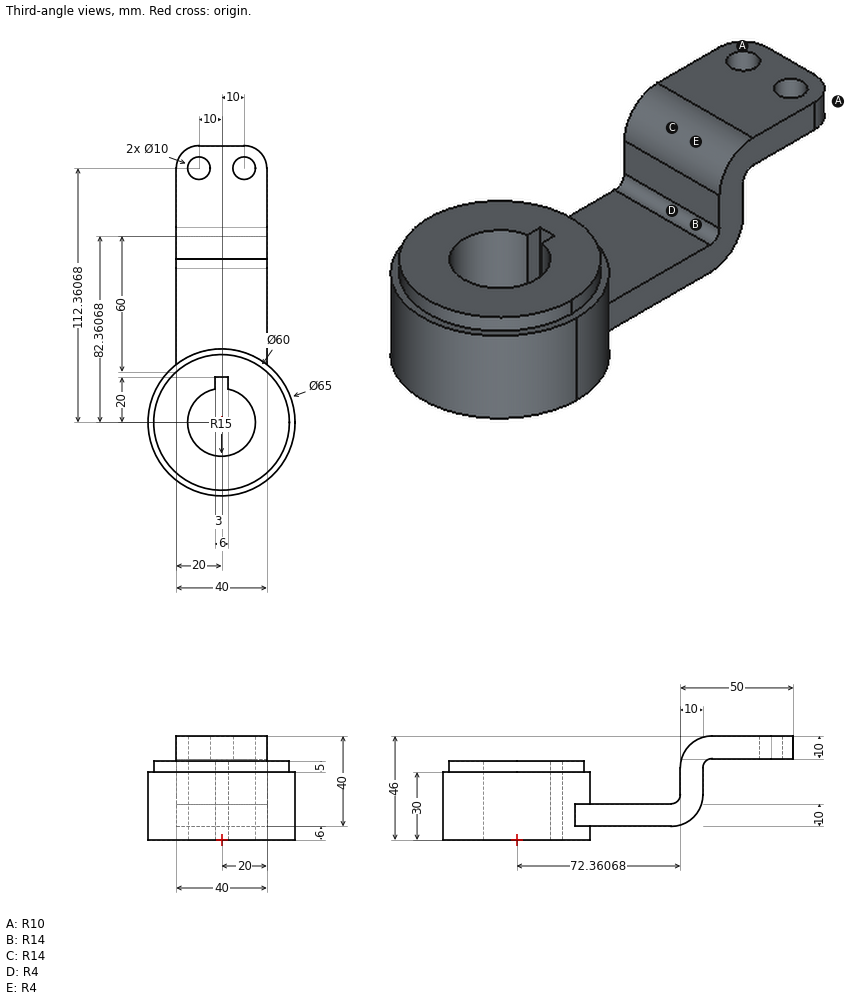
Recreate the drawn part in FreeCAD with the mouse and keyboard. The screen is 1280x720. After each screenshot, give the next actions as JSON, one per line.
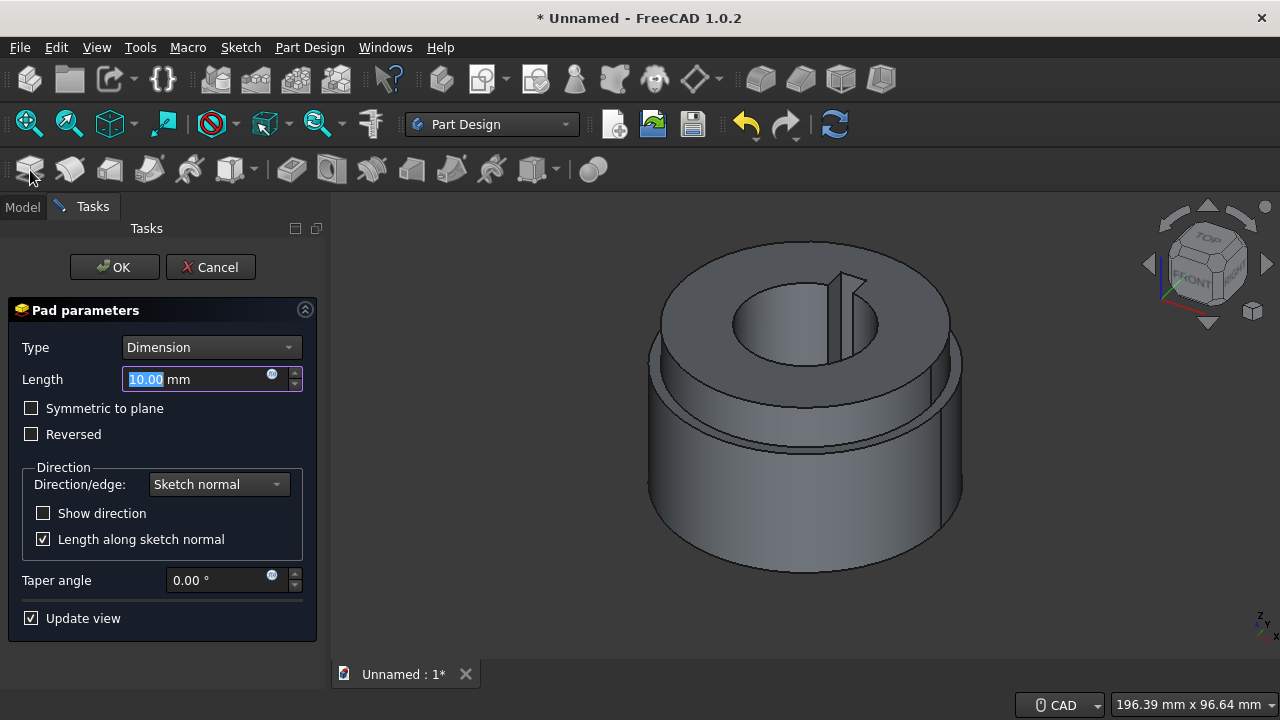
{"action": "type", "text": "5"}
{"action": "key", "text": "Tab"}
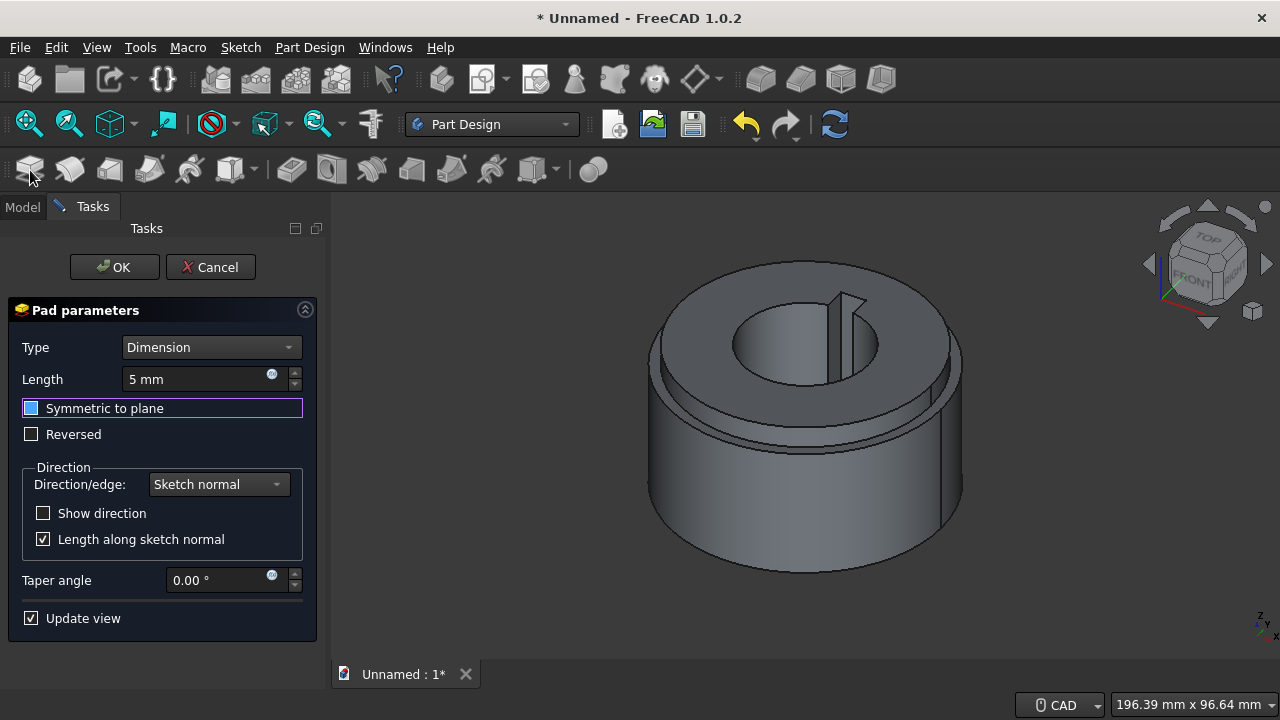
{"action": "left_click", "coordinate": [115, 267]}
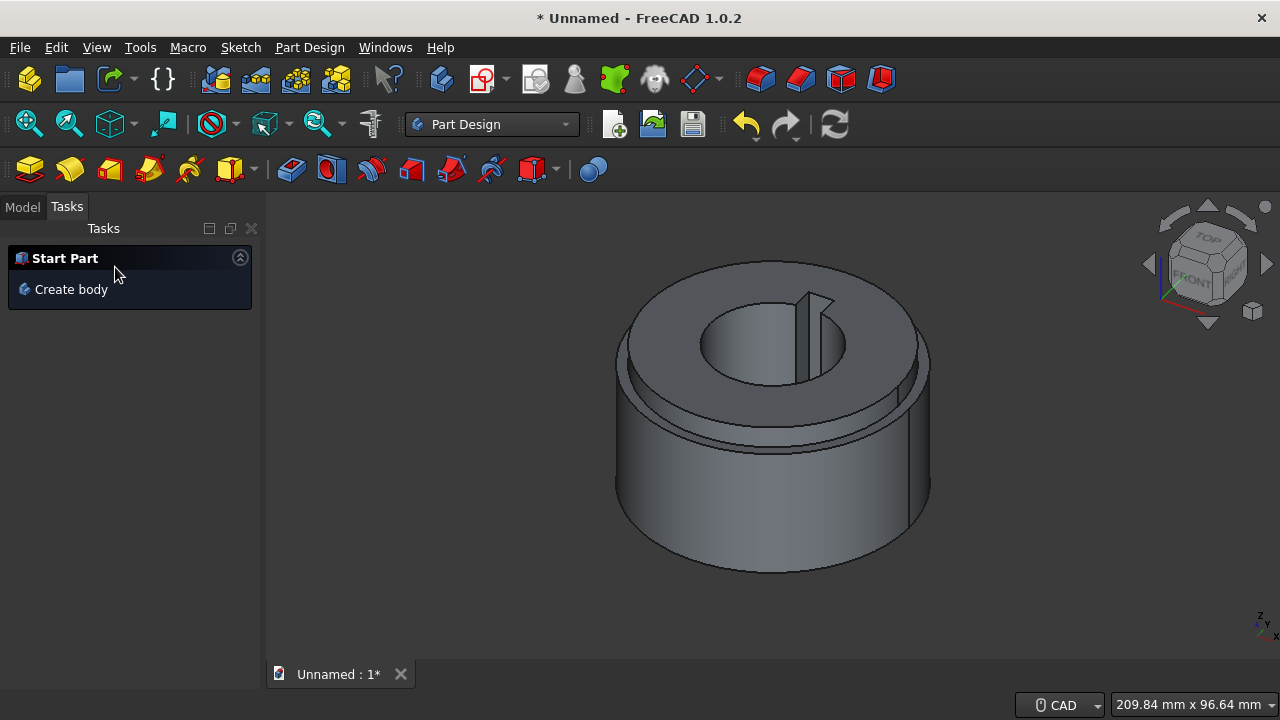
{"action": "left_click", "coordinate": [23, 206]}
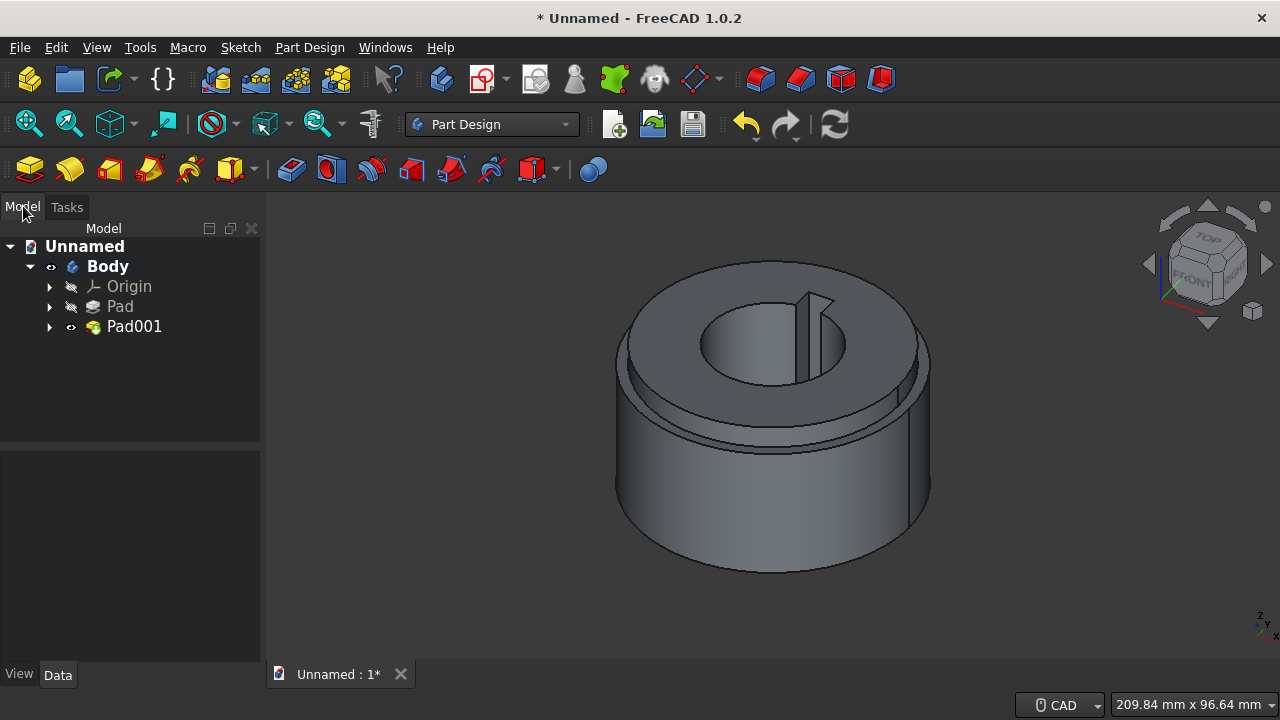
{"action": "left_click", "coordinate": [50, 287]}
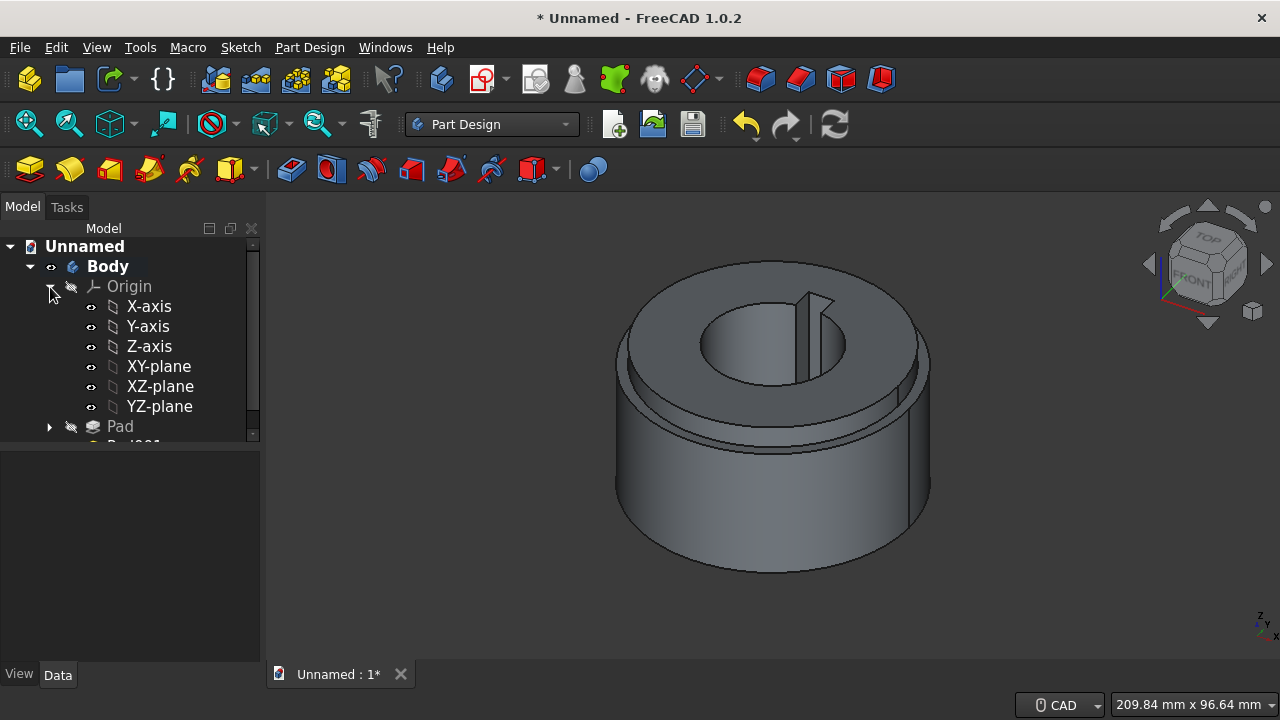
{"action": "left_click", "coordinate": [136, 367]}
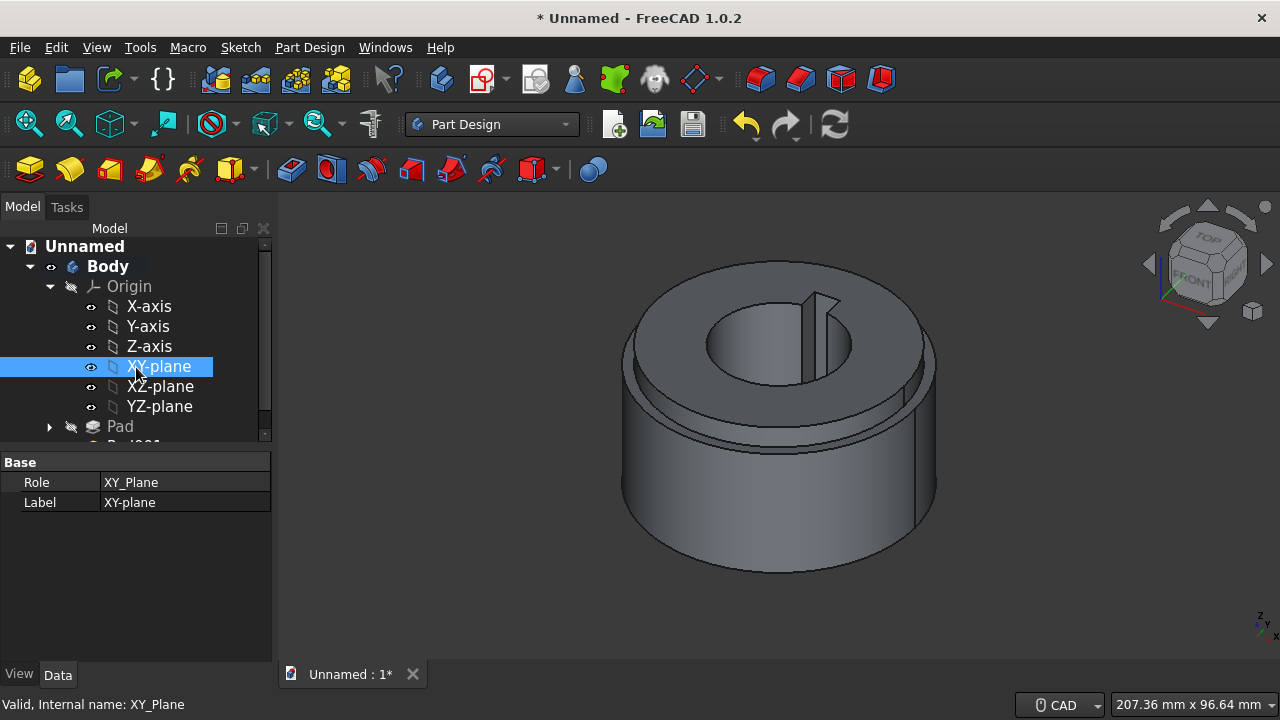
{"action": "left_click", "coordinate": [696, 80]}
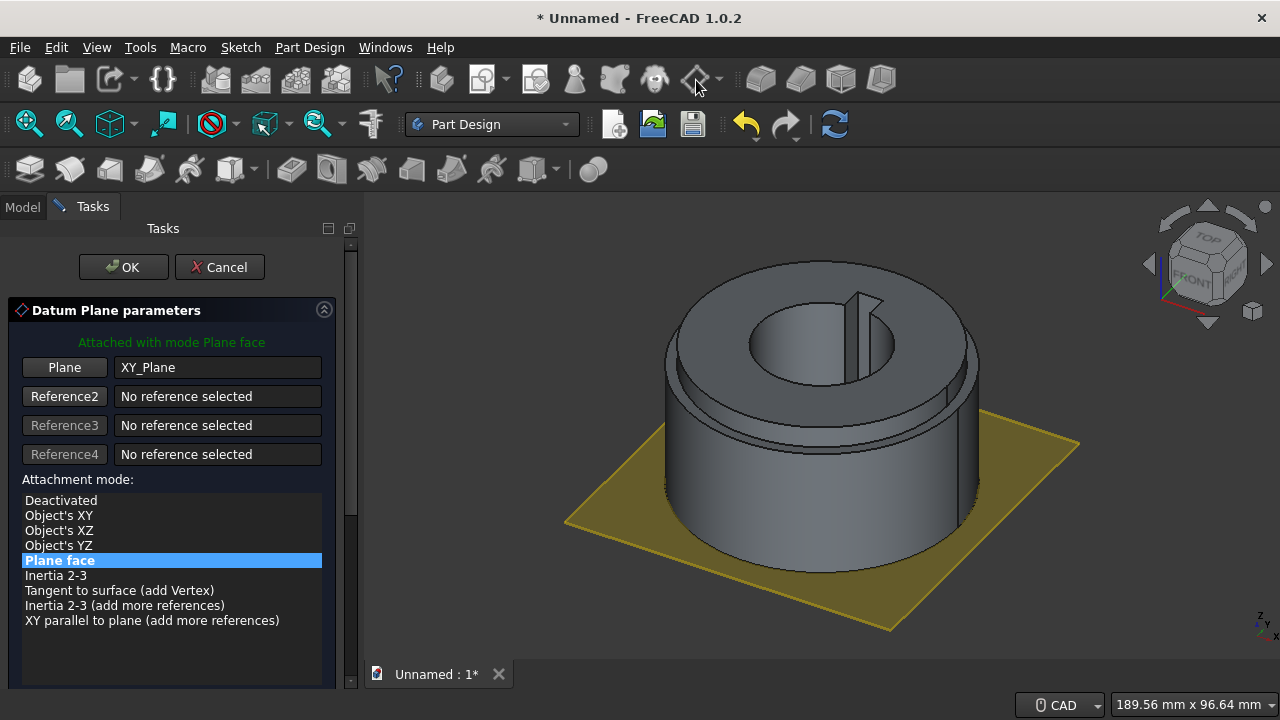
{"action": "scroll", "coordinate": [351, 463], "scroll_direction": "down", "scroll_amount": 3}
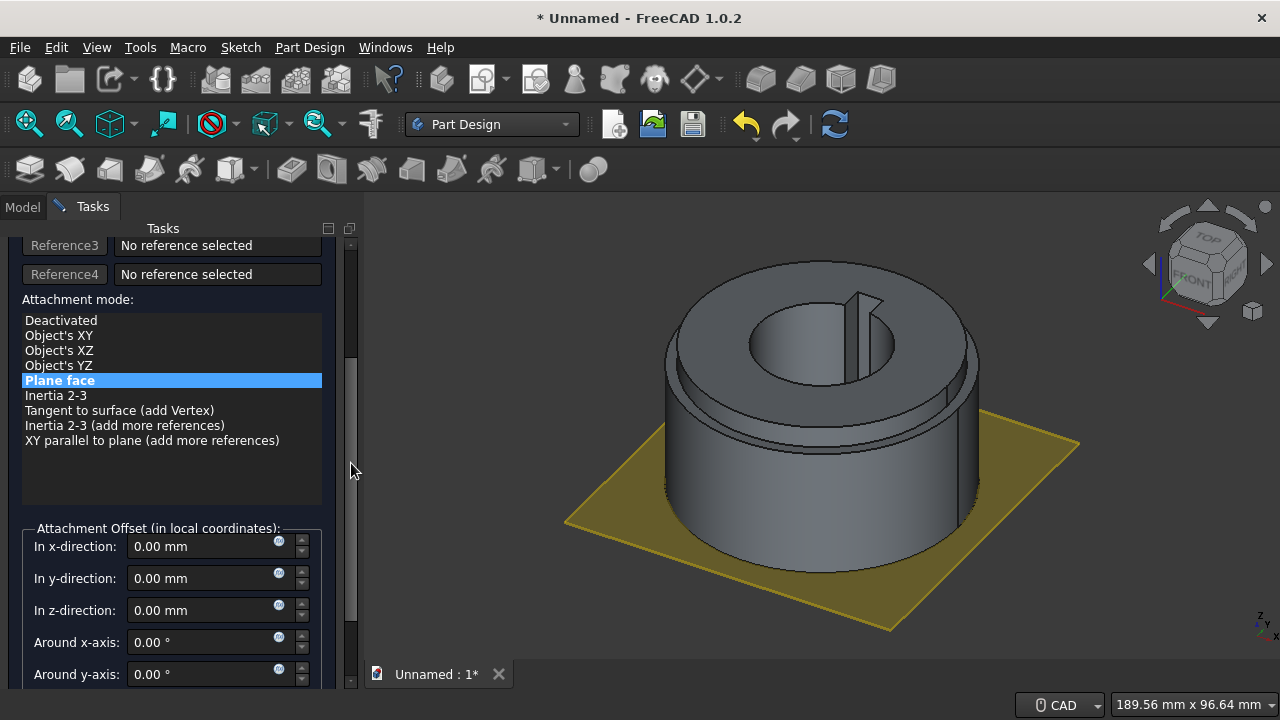
{"action": "triple_click", "coordinate": [210, 610]}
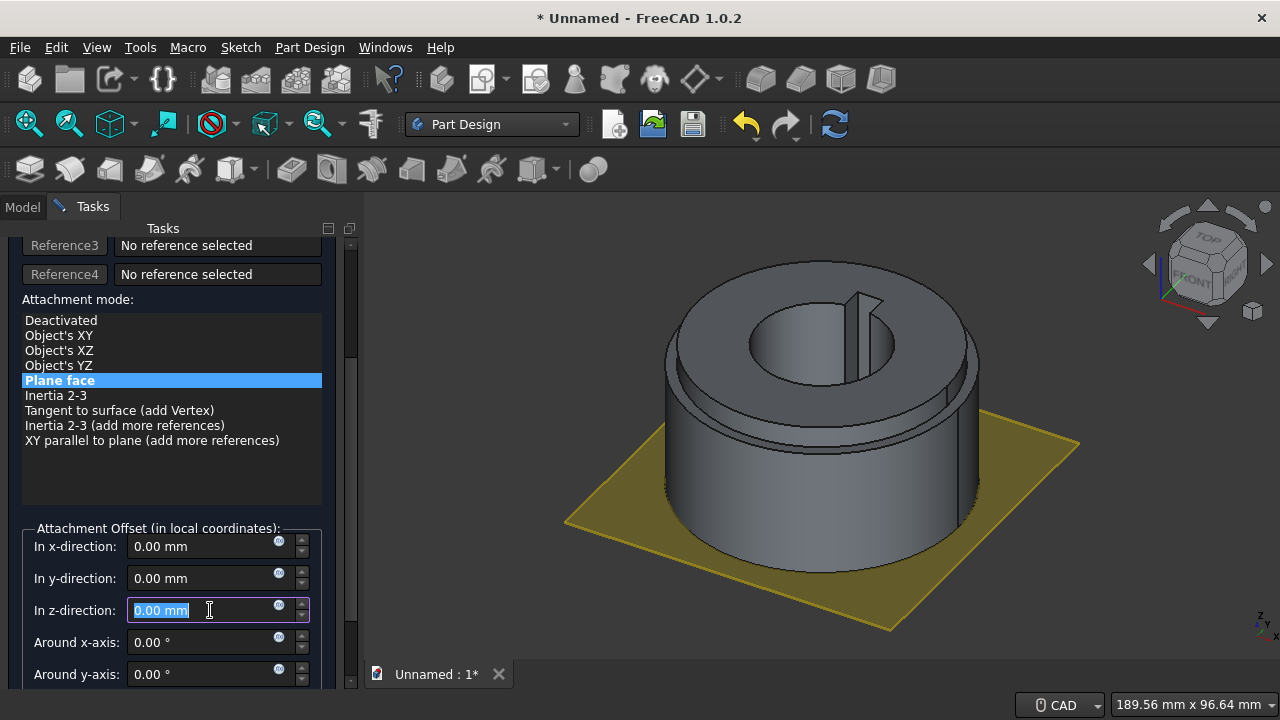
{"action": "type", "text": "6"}
{"action": "key", "text": "Tab"}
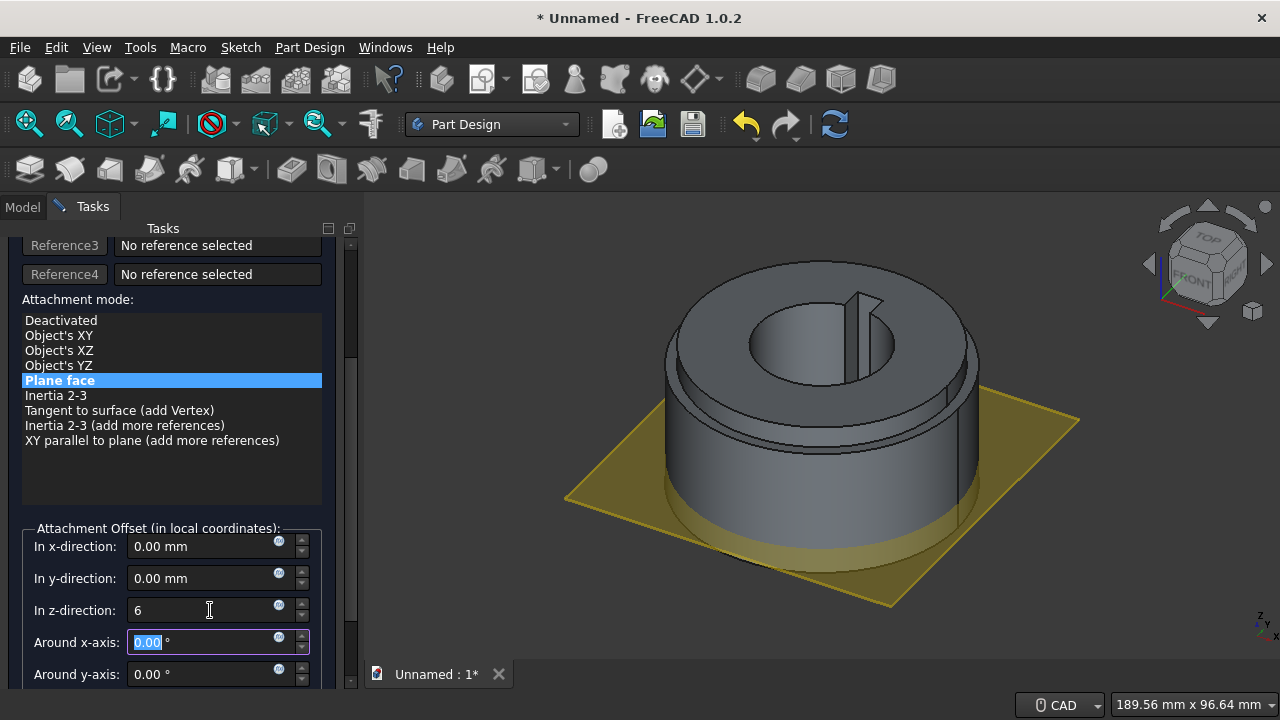
{"action": "scroll", "coordinate": [351, 463], "scroll_direction": "up", "scroll_amount": 4}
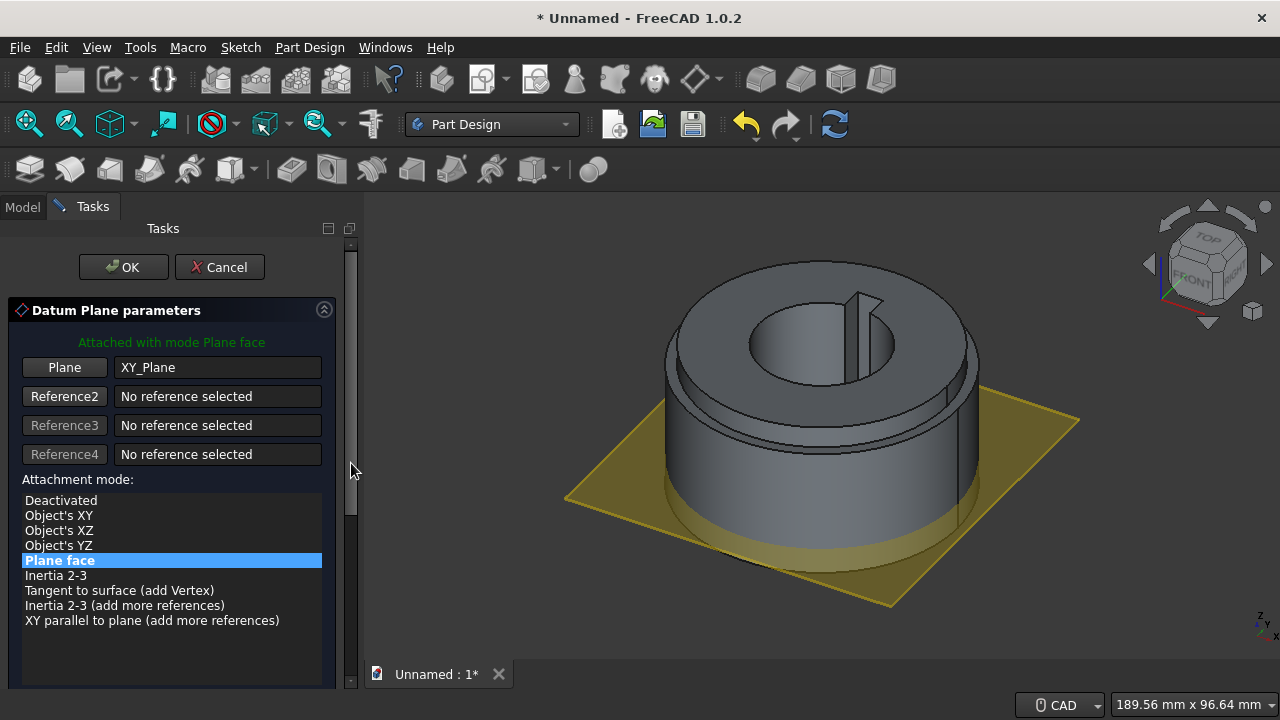
{"action": "left_click", "coordinate": [124, 267]}